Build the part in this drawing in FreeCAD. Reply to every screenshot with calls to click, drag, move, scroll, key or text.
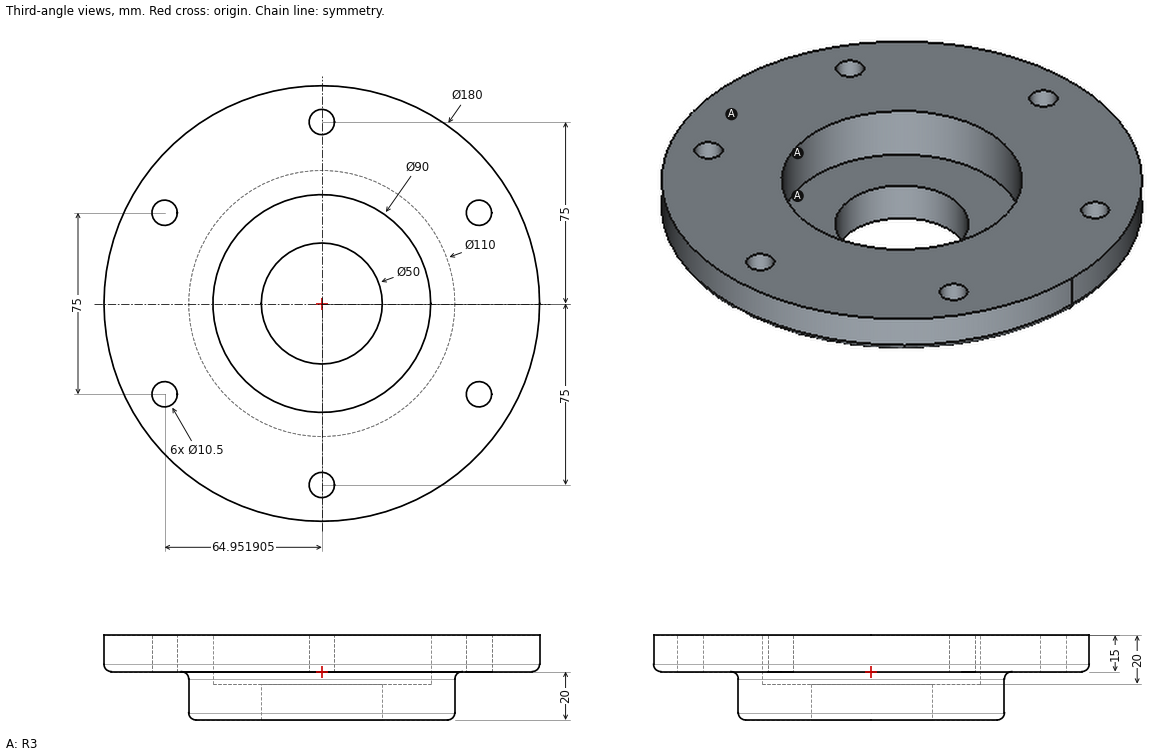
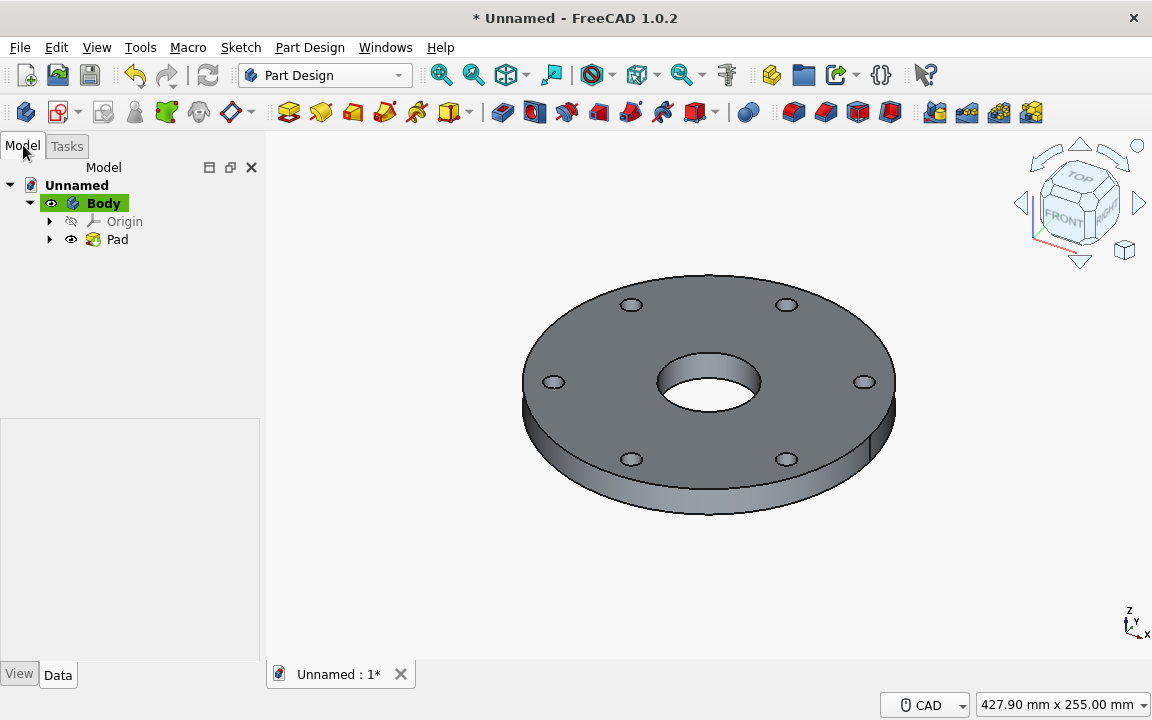
click(50, 221)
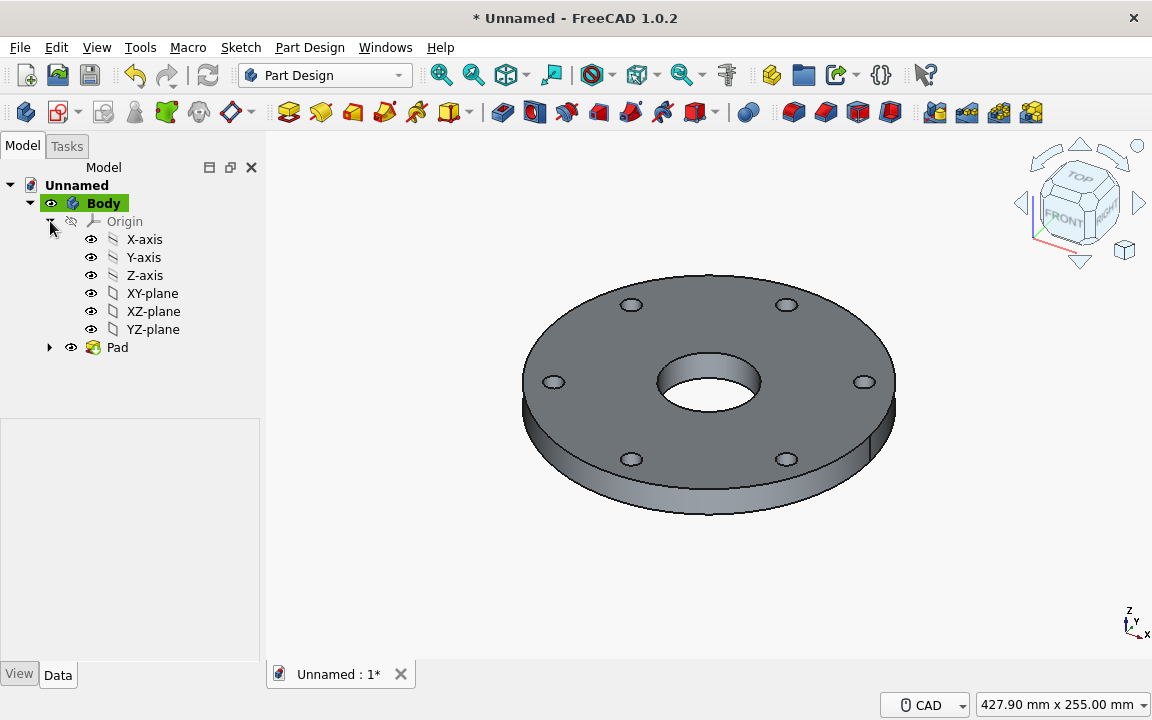
click(136, 293)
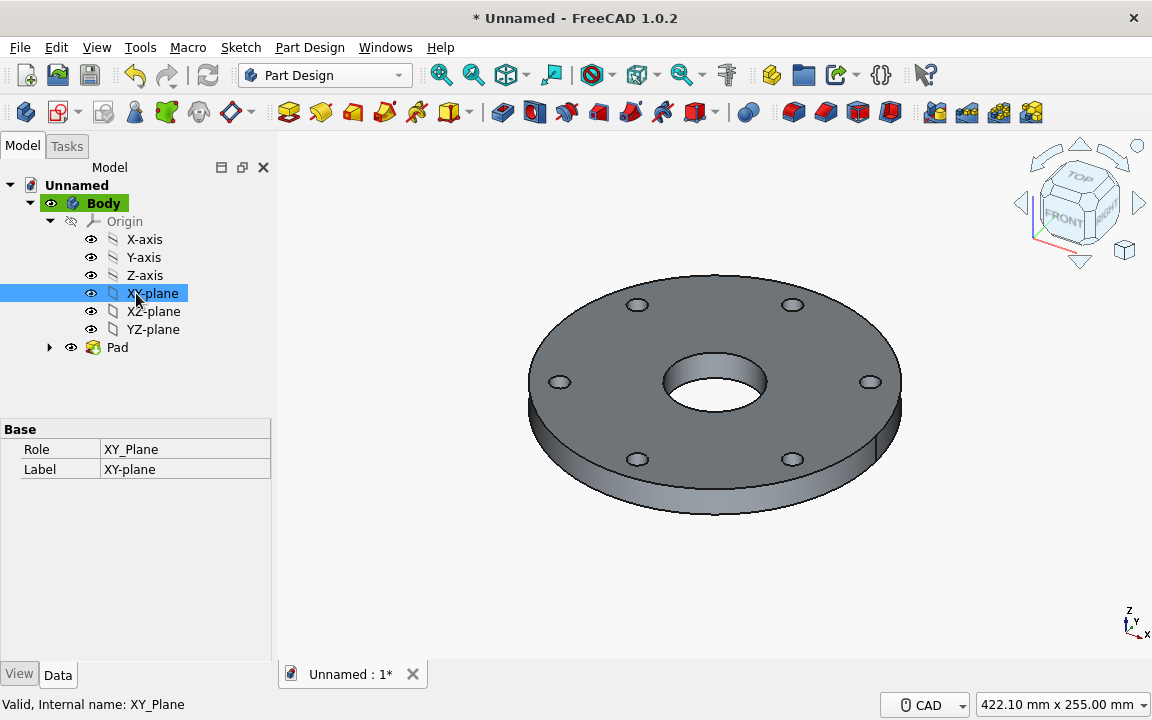
click(232, 112)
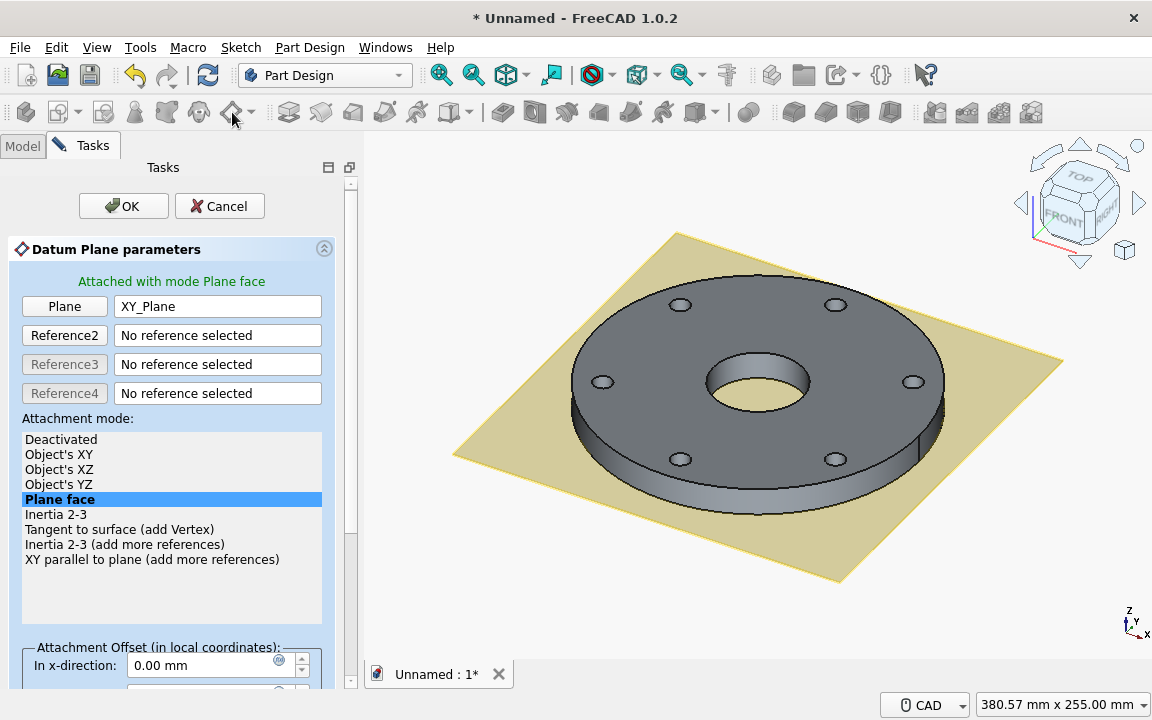
scroll(351, 432, down, 2)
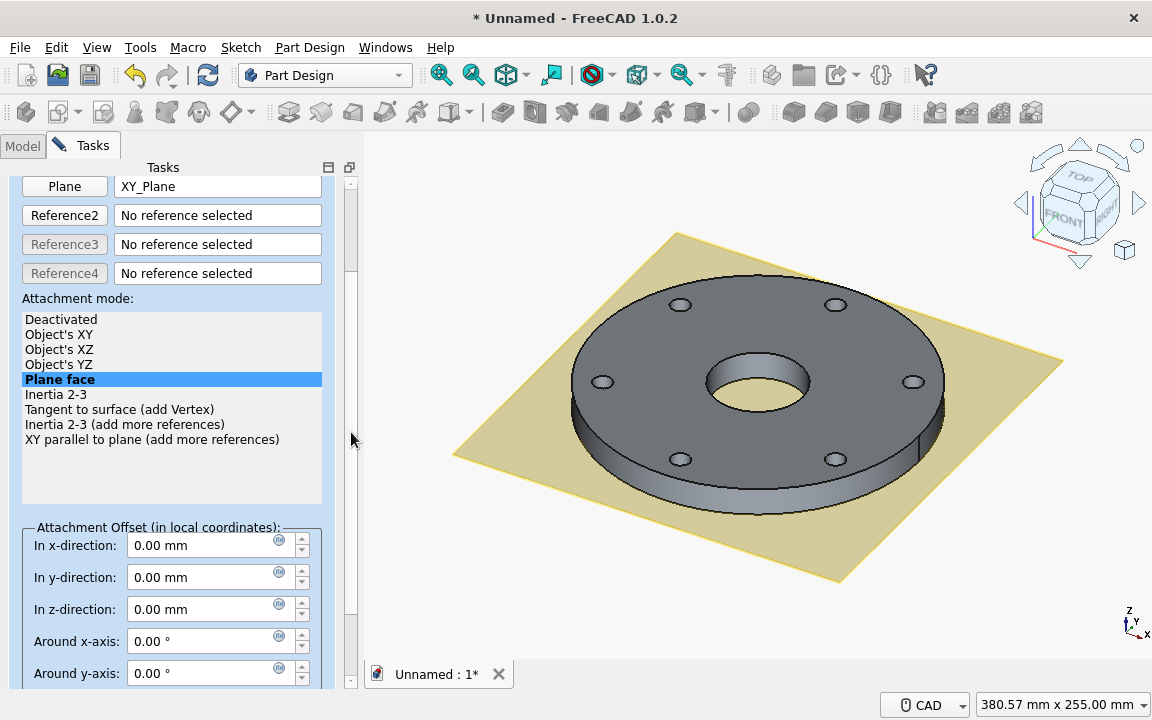
triple_click(210, 609)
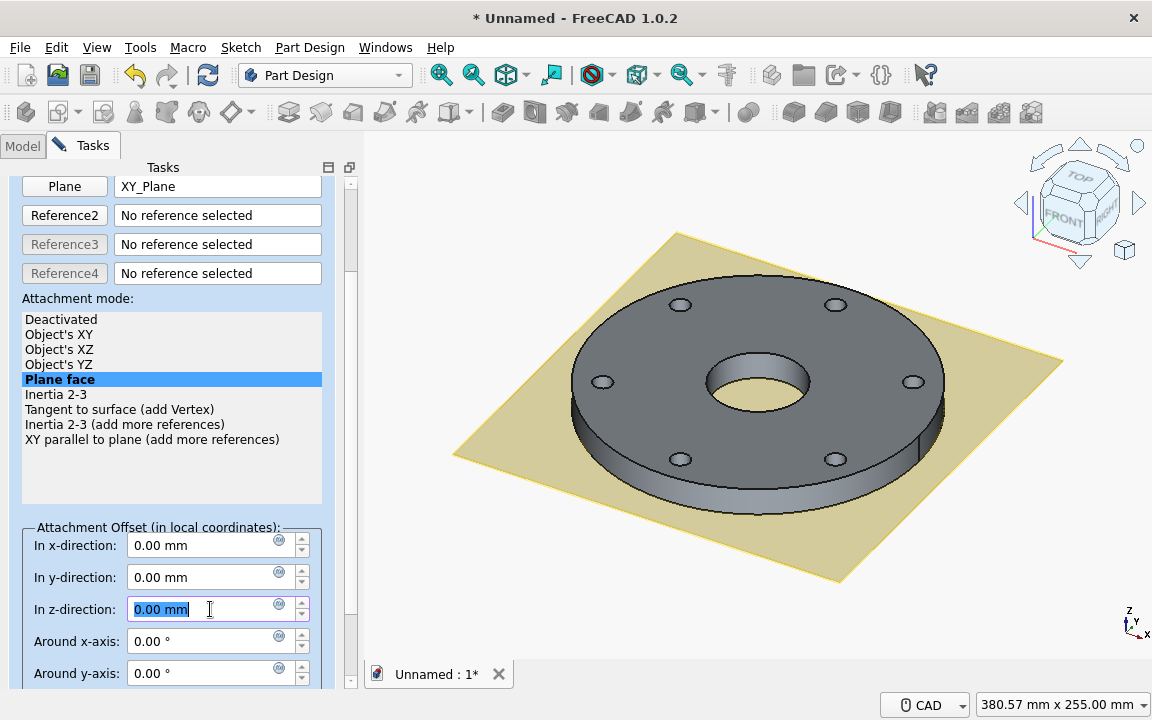
text(-20)
key(Tab)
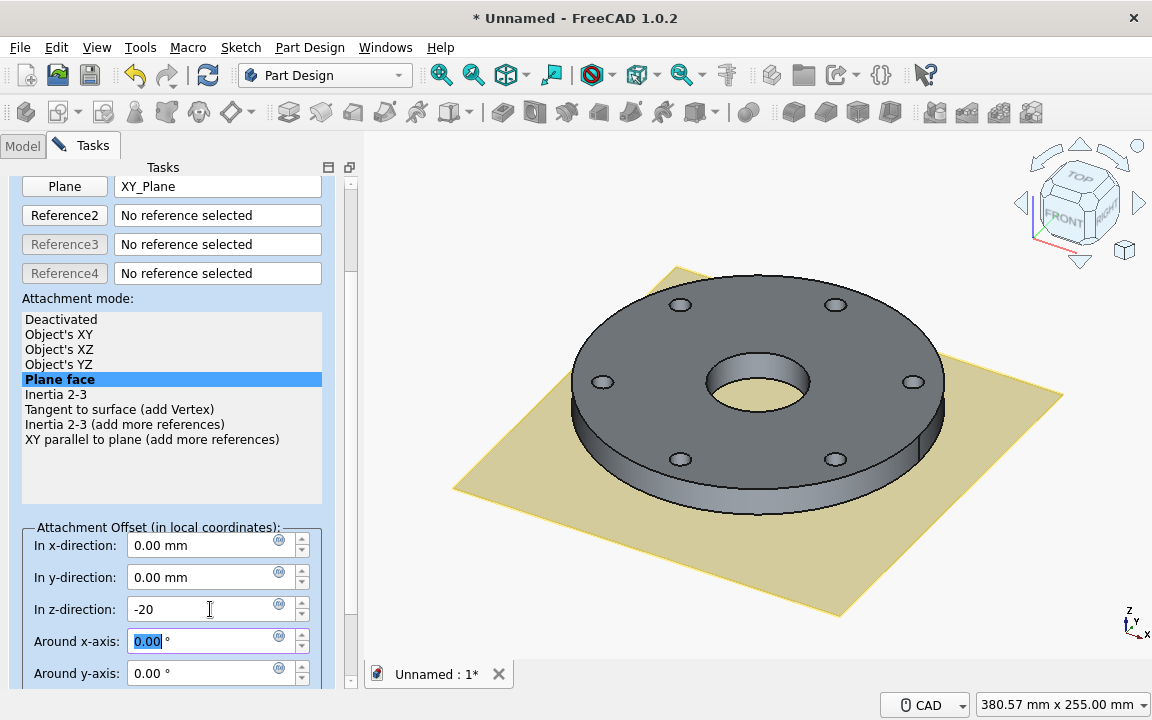
scroll(351, 432, up, 3)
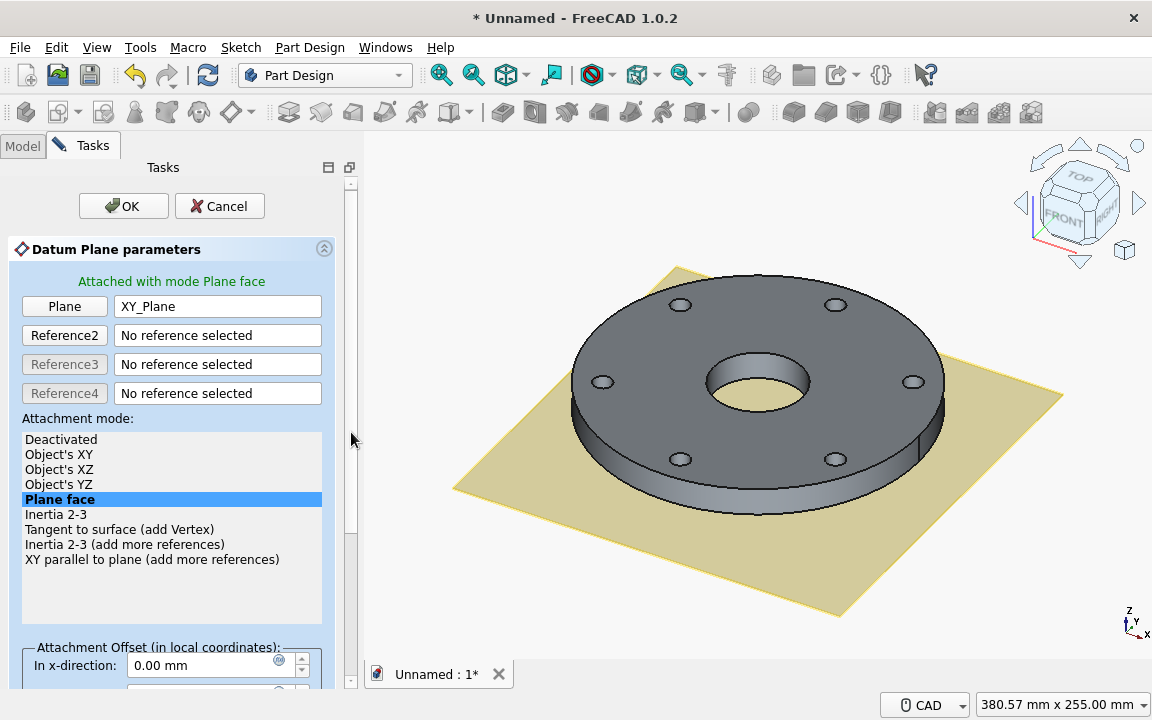
click(124, 206)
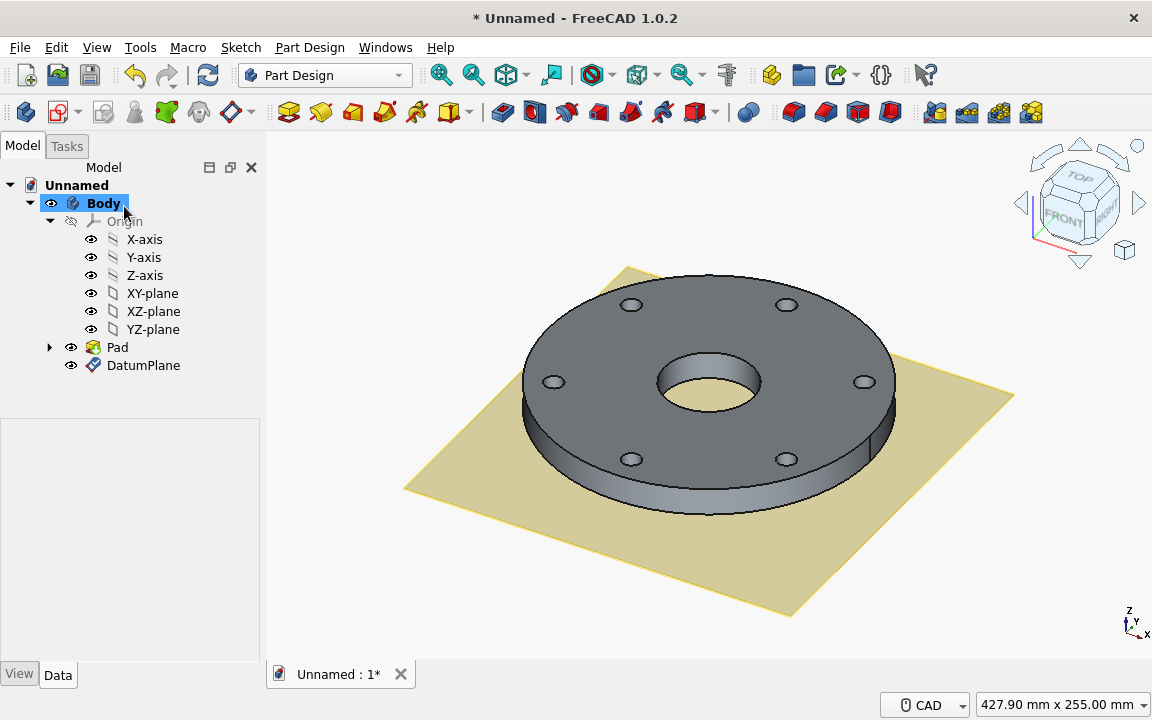
click(116, 365)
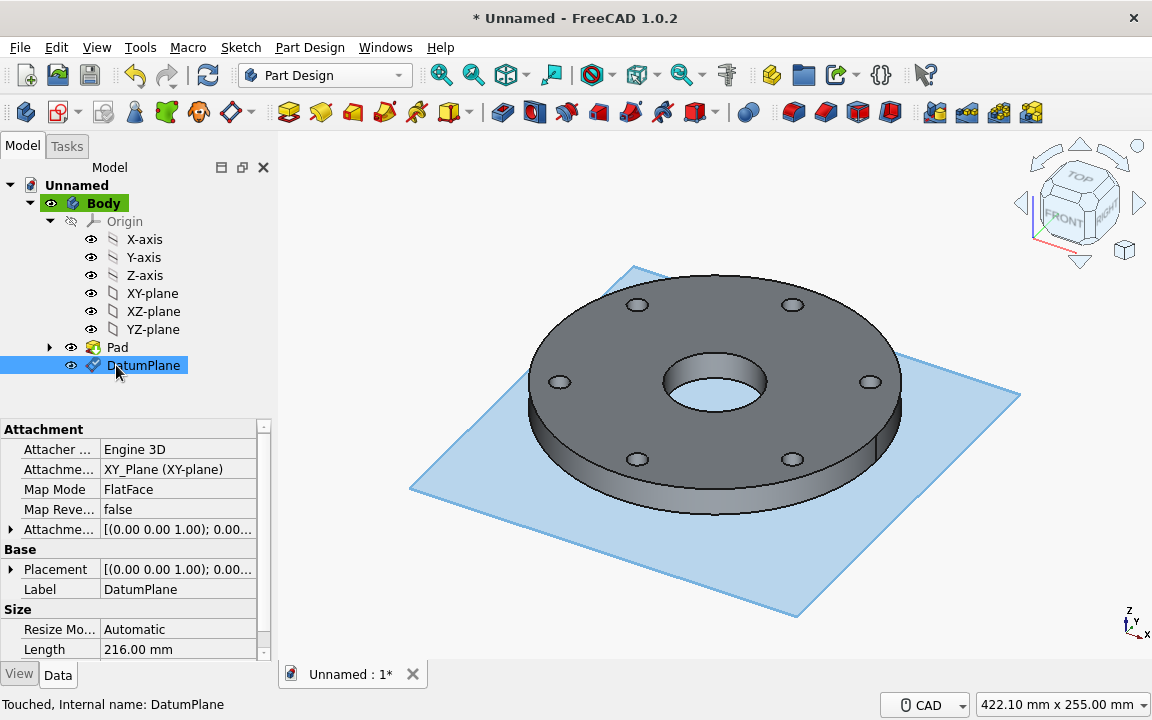
click(58, 112)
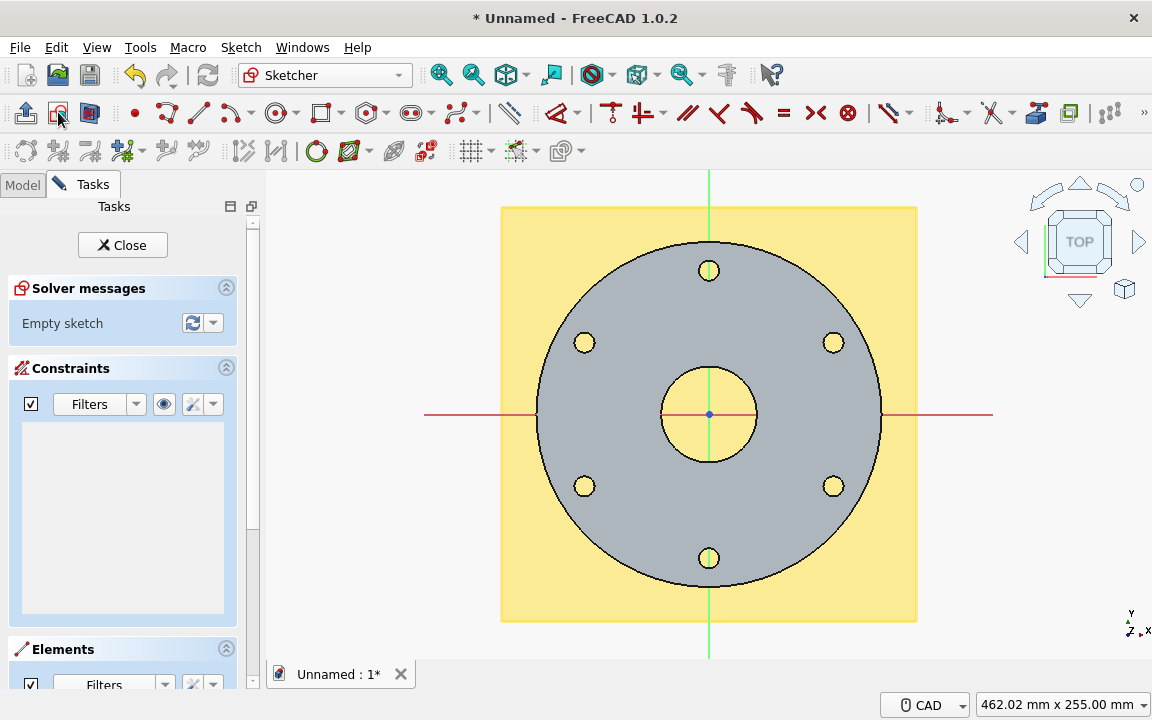
key(q)
key(s)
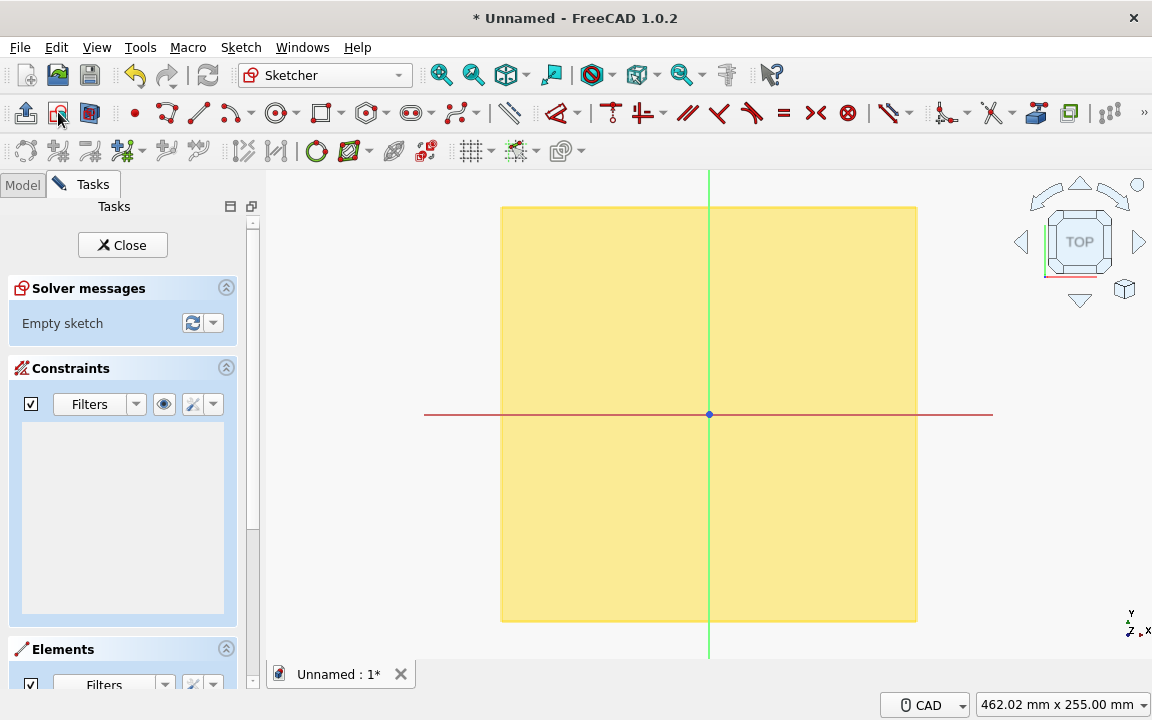
scroll(848, 414, up, 2)